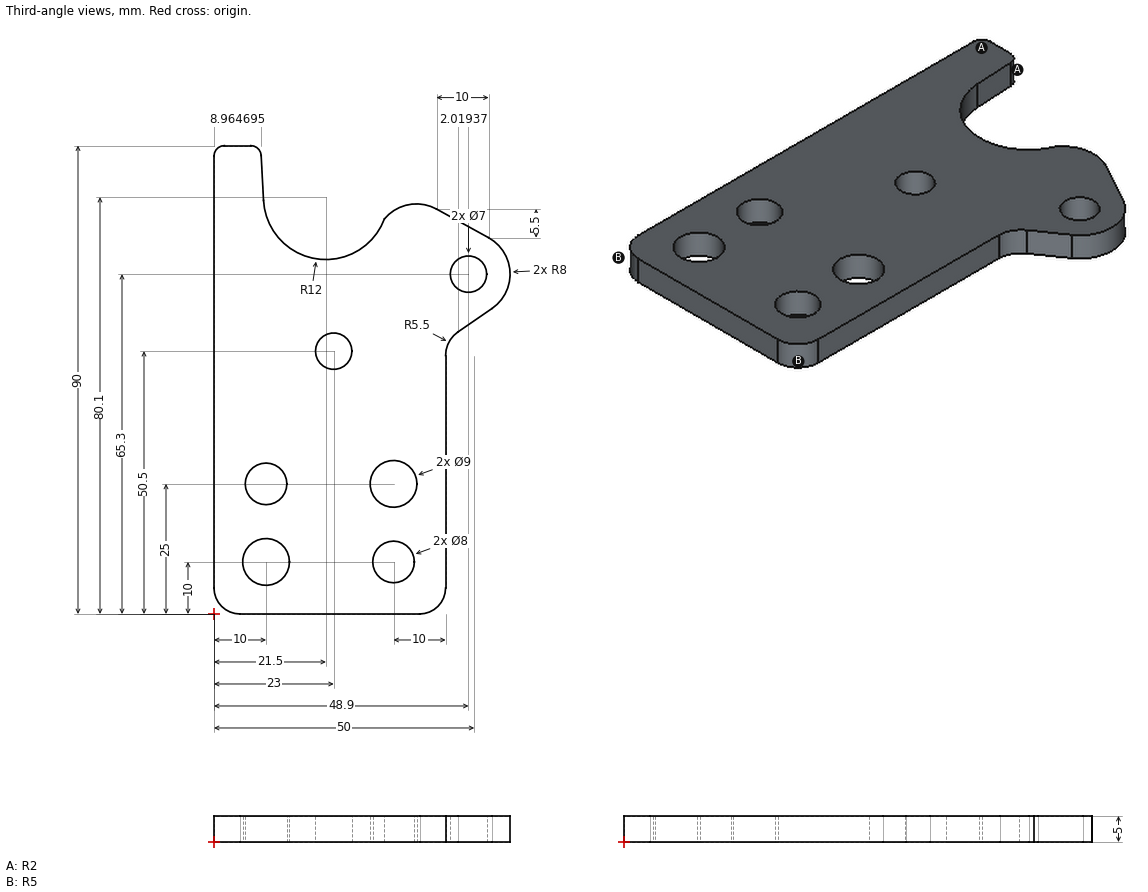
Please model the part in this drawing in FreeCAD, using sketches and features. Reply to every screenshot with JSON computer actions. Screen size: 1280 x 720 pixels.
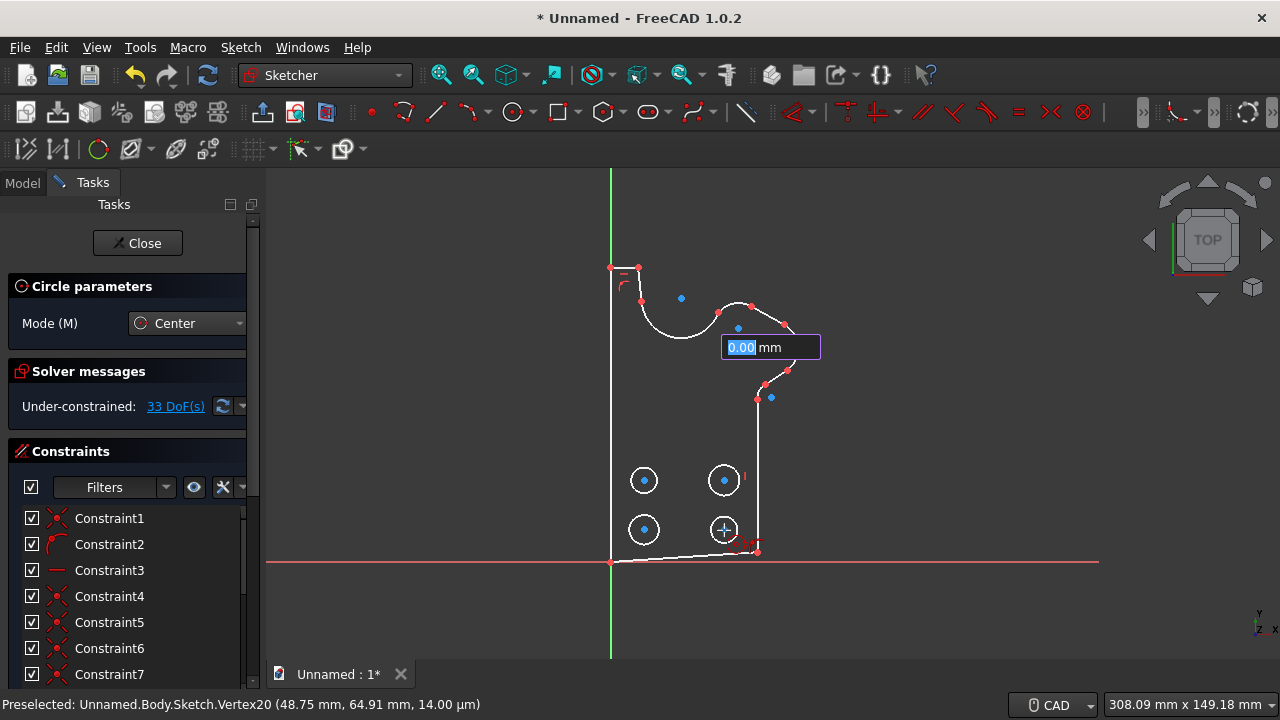
{"action": "scroll", "coordinate": [780, 339], "scroll_direction": "up", "scroll_amount": 2}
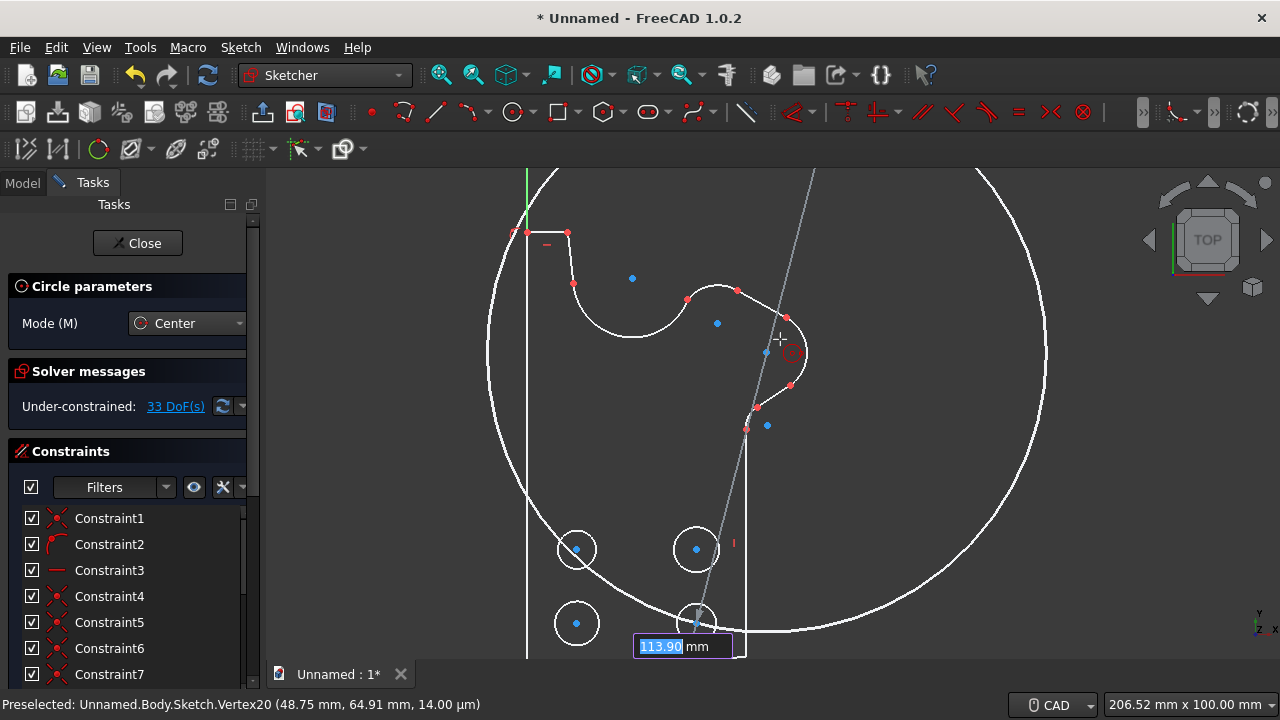
{"action": "left_click", "coordinate": [780, 339]}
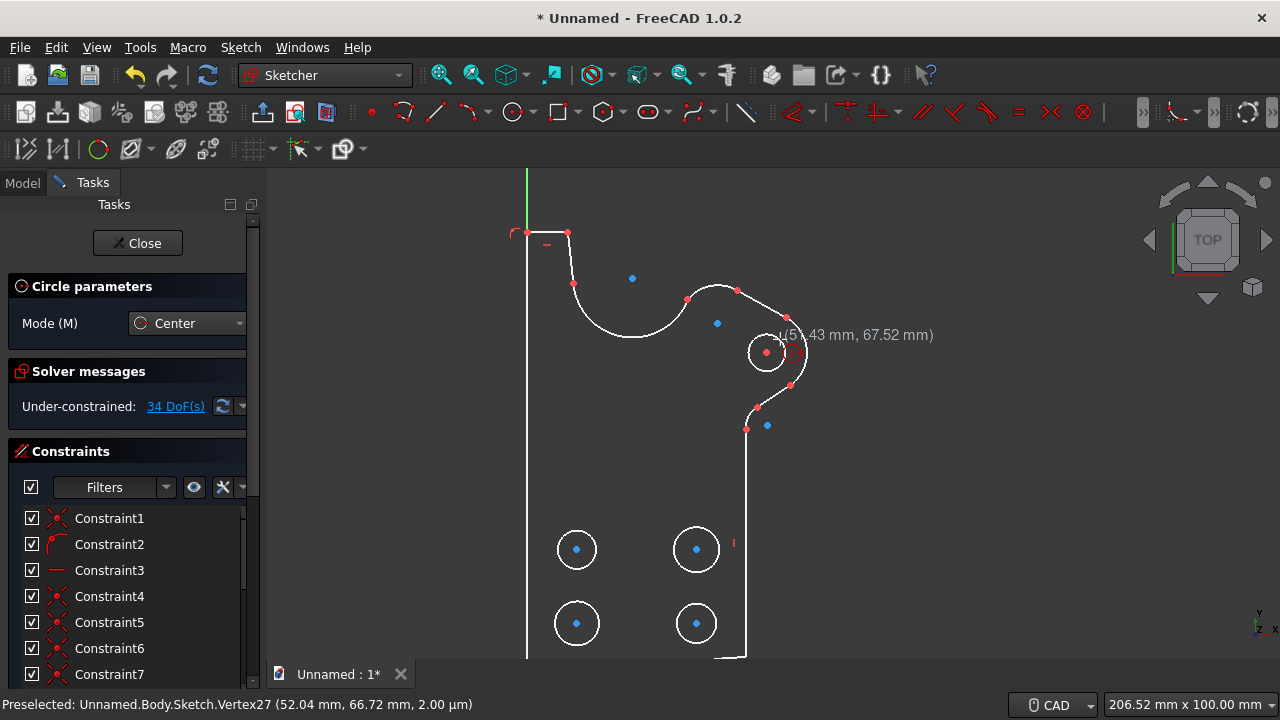
{"action": "scroll", "coordinate": [640, 424], "scroll_direction": "up", "scroll_amount": 2}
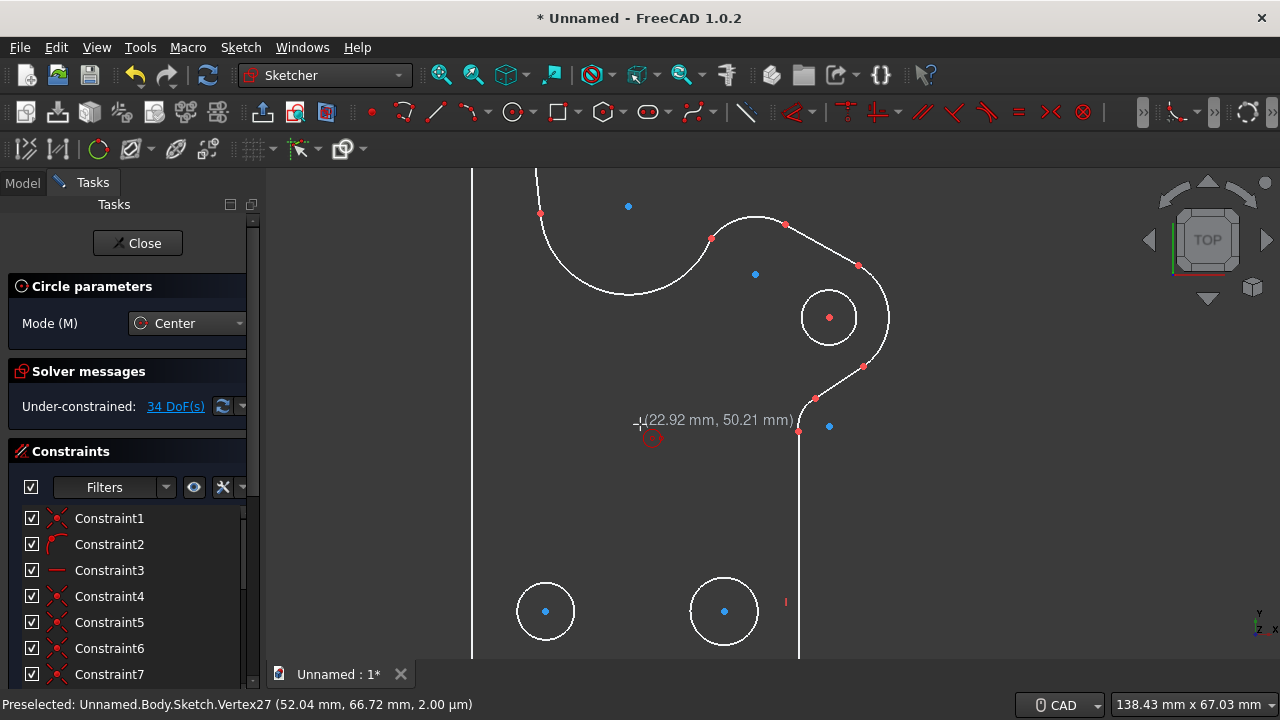
{"action": "left_click", "coordinate": [640, 423]}
{"action": "left_click", "coordinate": [659, 405]}
{"action": "key", "text": "Escape"}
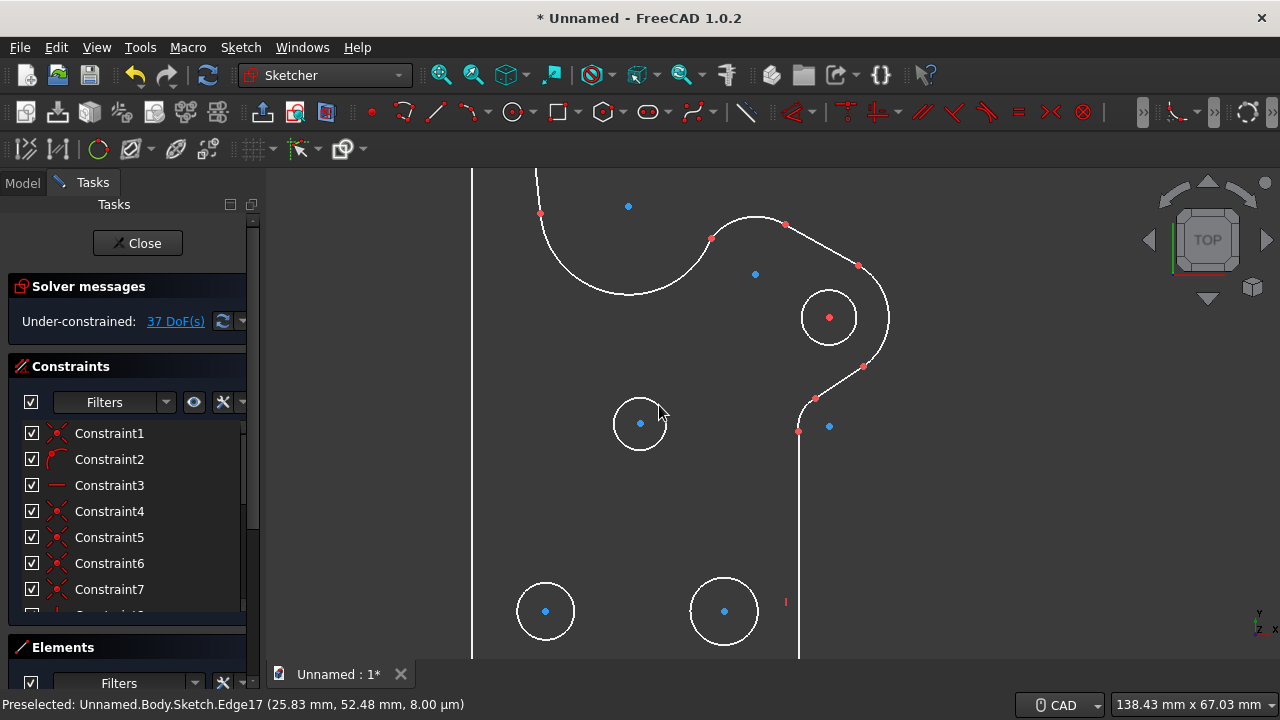
{"action": "left_click", "coordinate": [539, 199]}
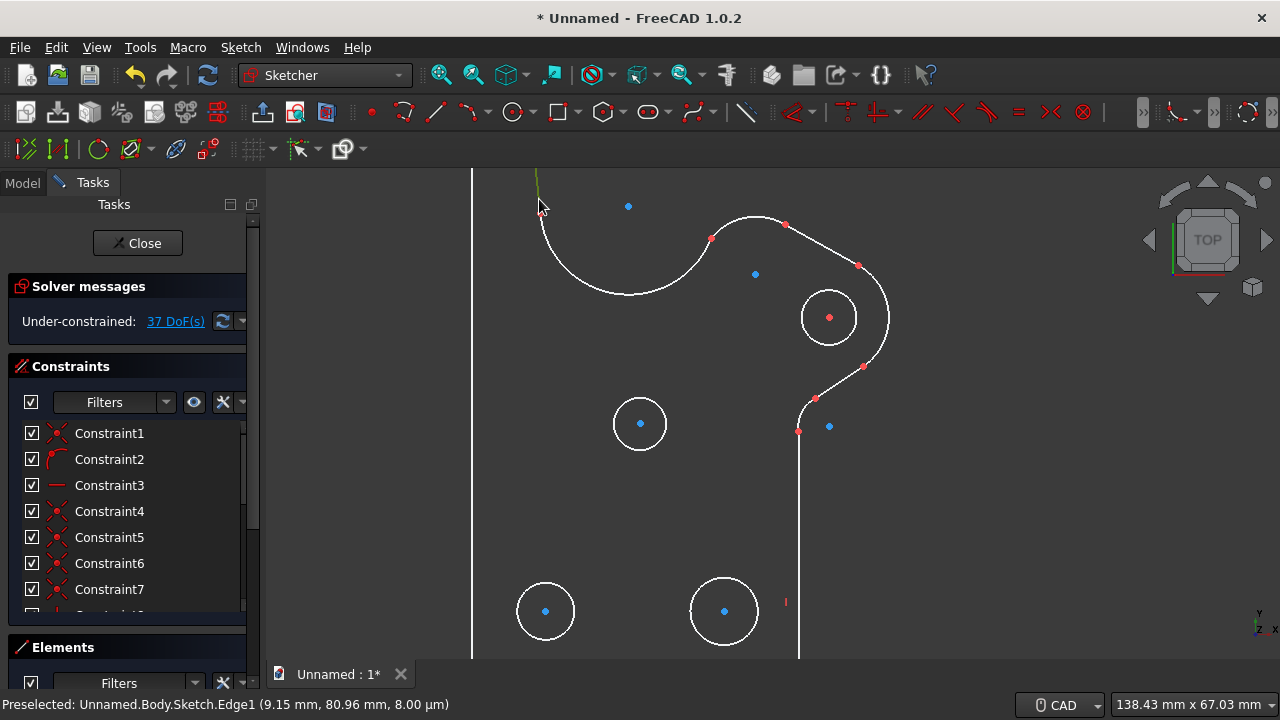
{"action": "left_click", "coordinate": [573, 275]}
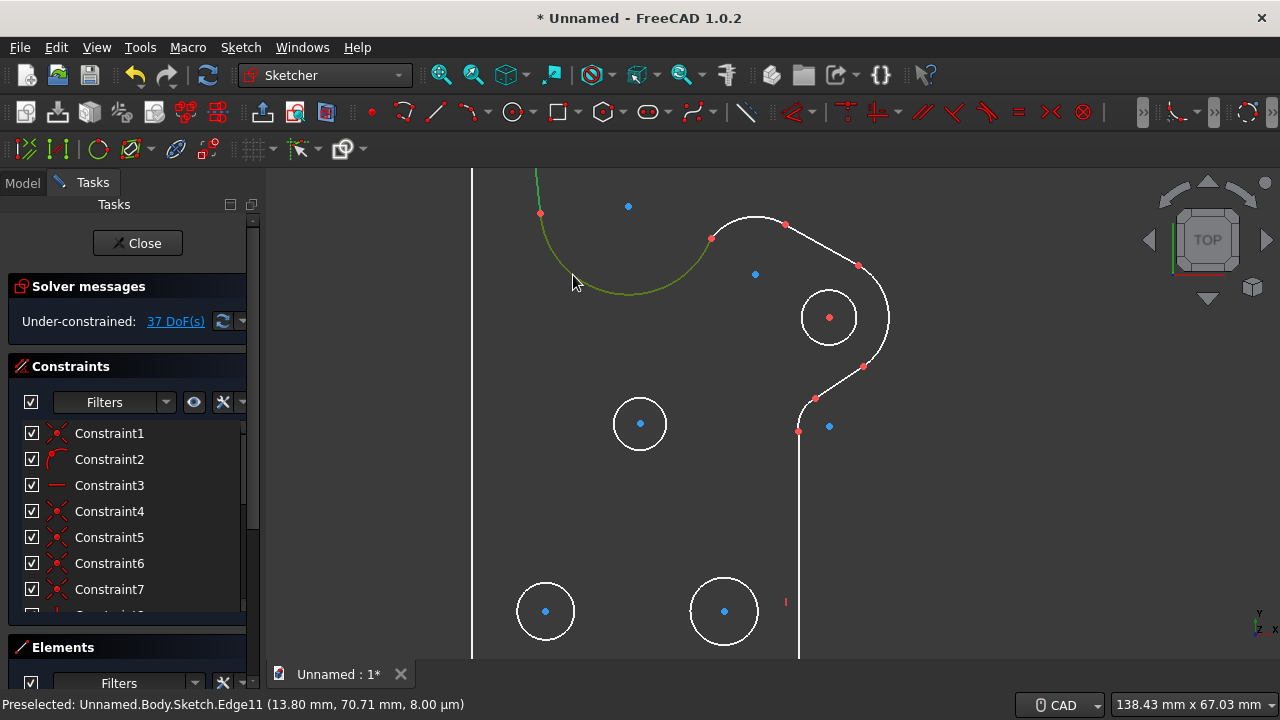
{"action": "key", "text": "t"}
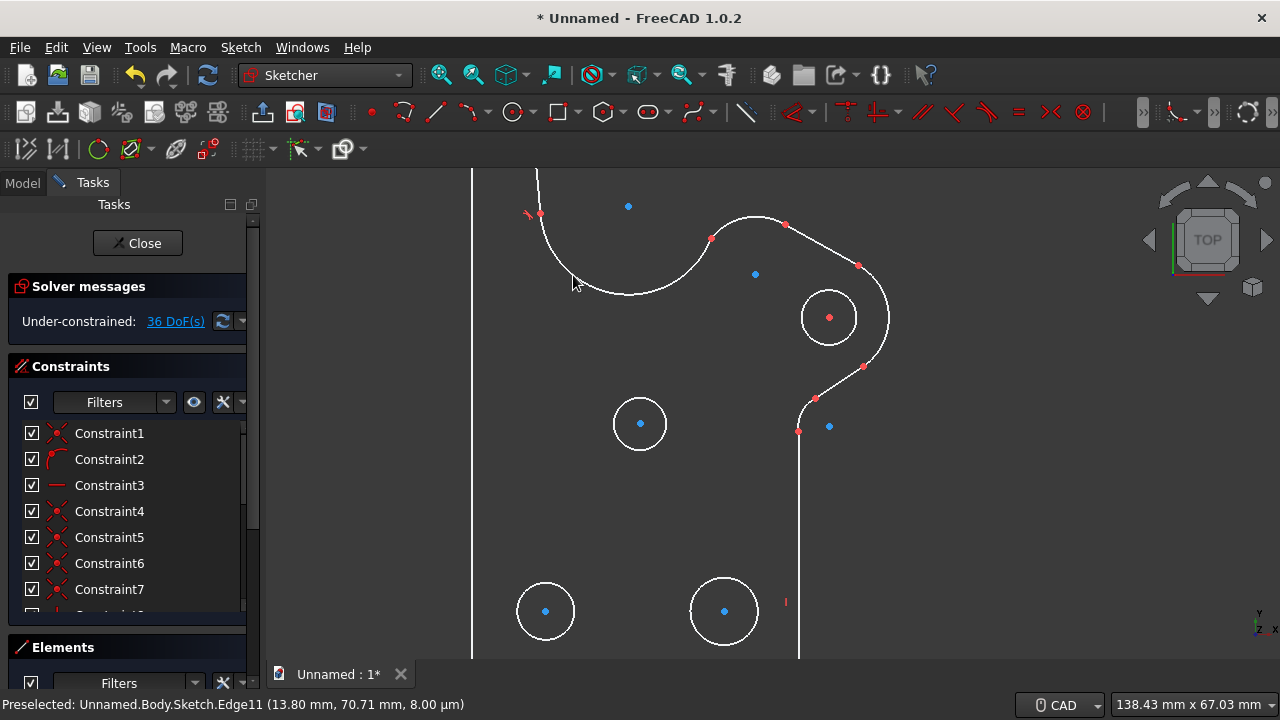
{"action": "left_click", "coordinate": [799, 533]}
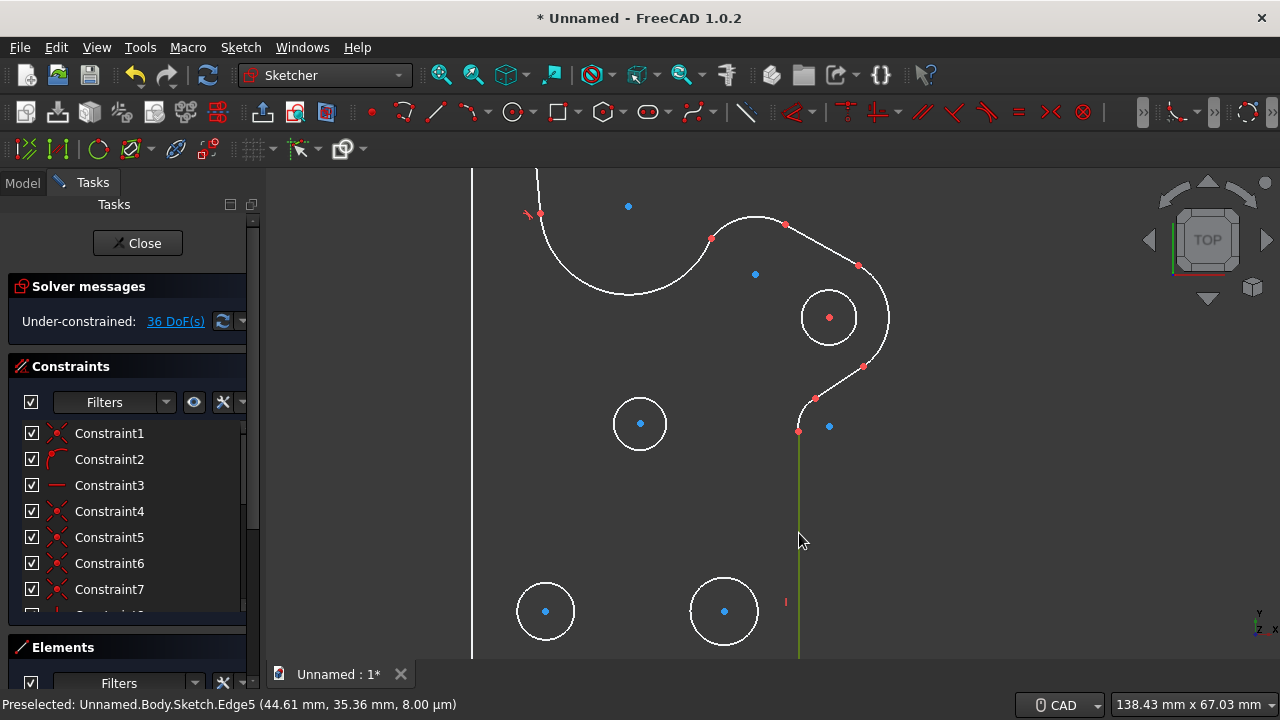
{"action": "left_click", "coordinate": [806, 406]}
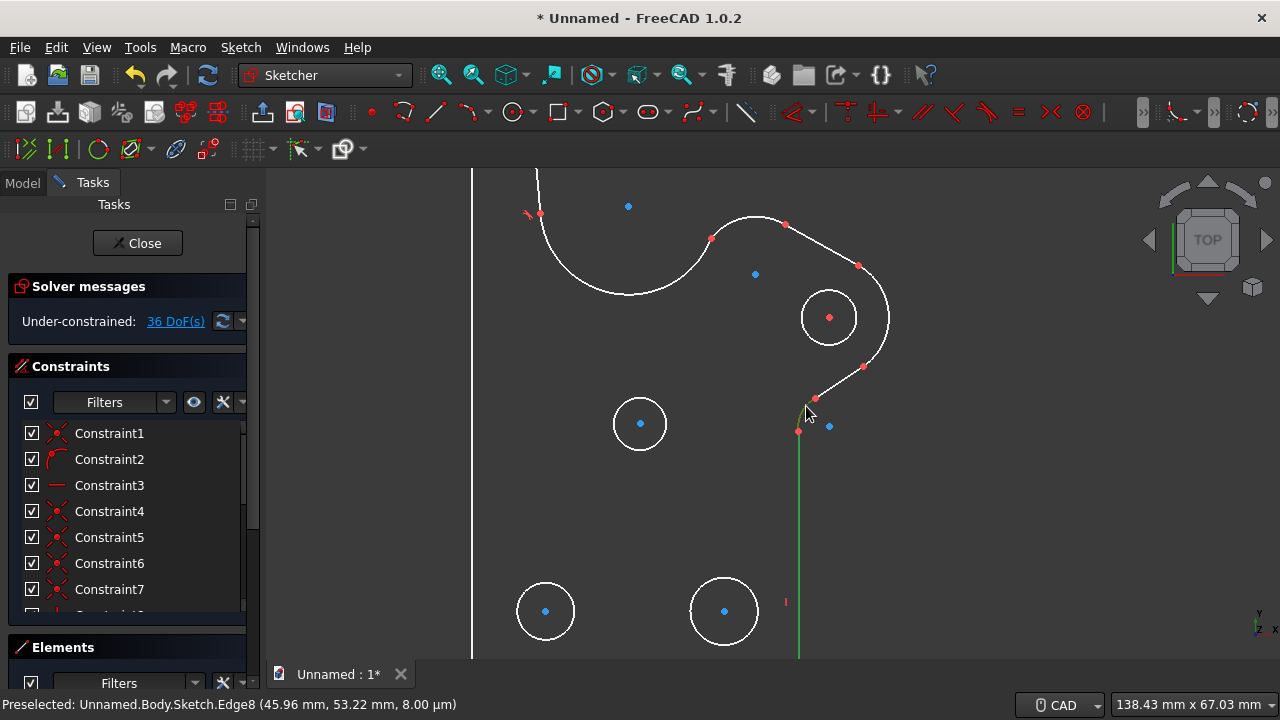
{"action": "key", "text": "t"}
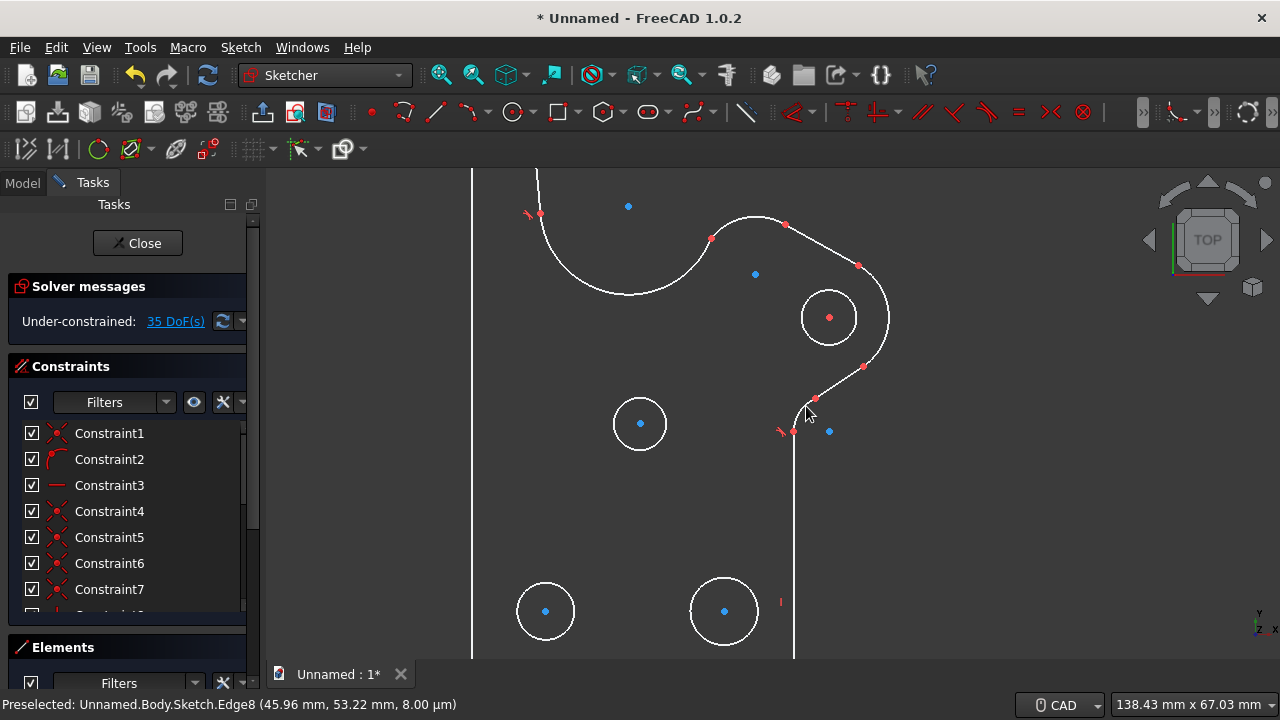
{"action": "left_click", "coordinate": [830, 389]}